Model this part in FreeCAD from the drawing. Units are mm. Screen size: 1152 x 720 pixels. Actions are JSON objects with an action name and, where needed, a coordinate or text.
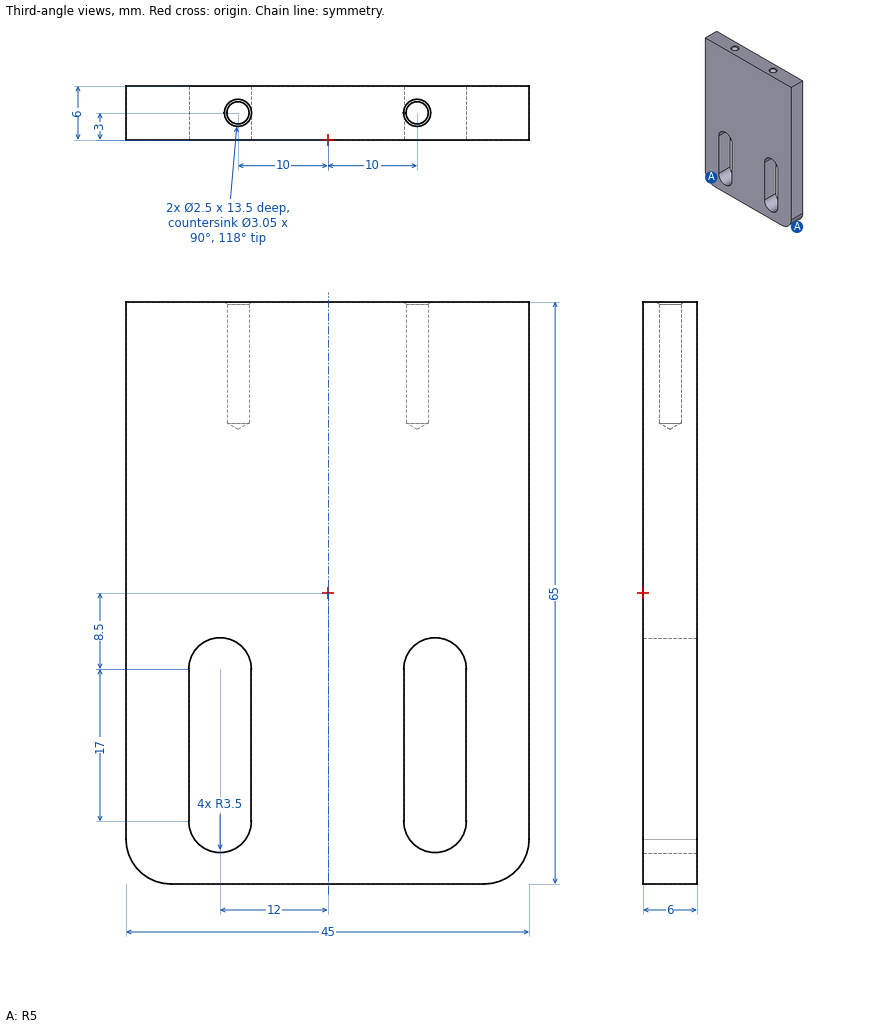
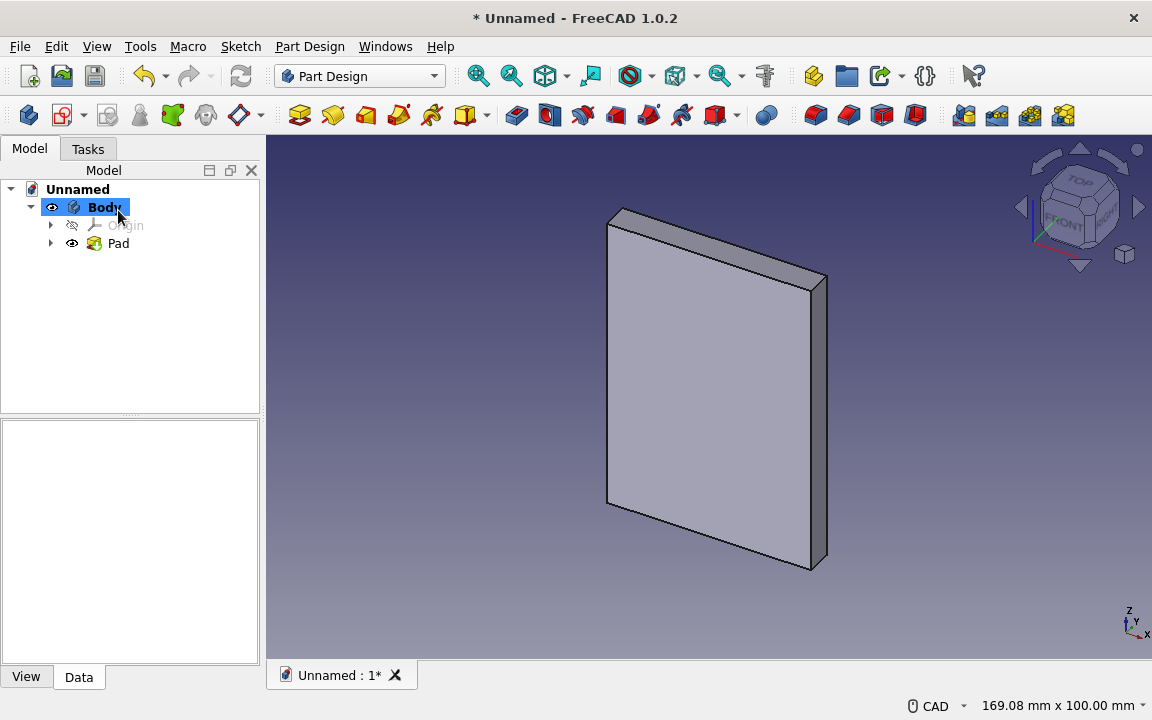
{"action": "key", "text": "4"}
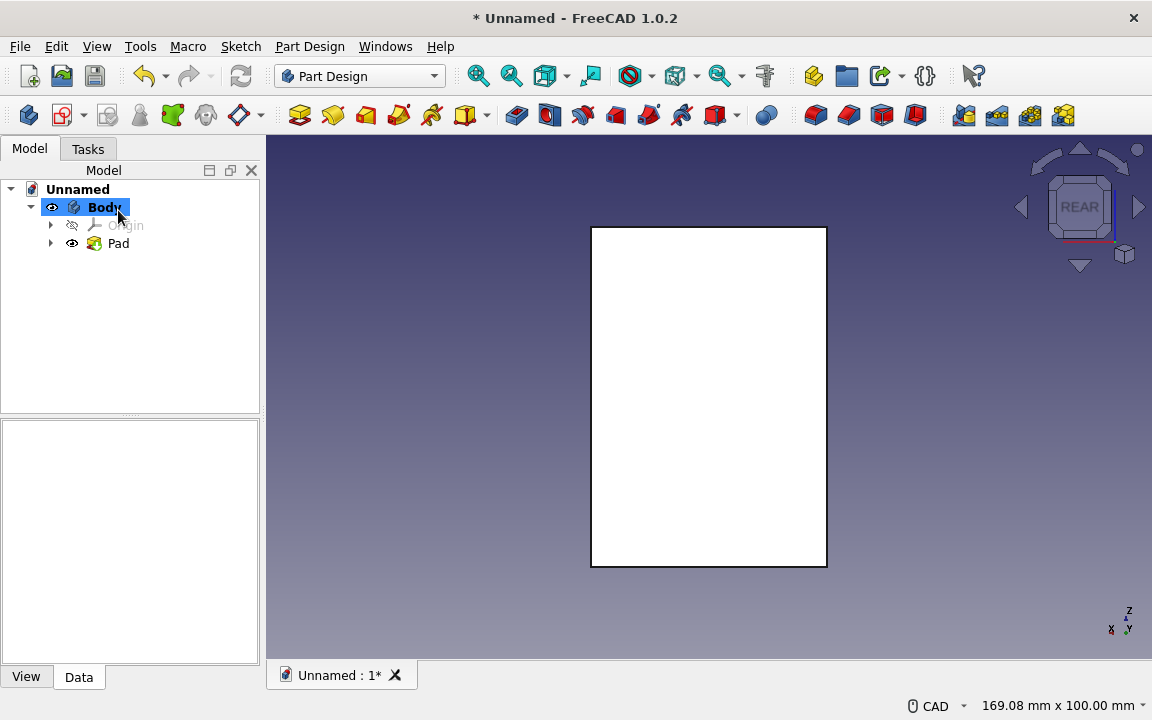
{"action": "left_click", "coordinate": [709, 347]}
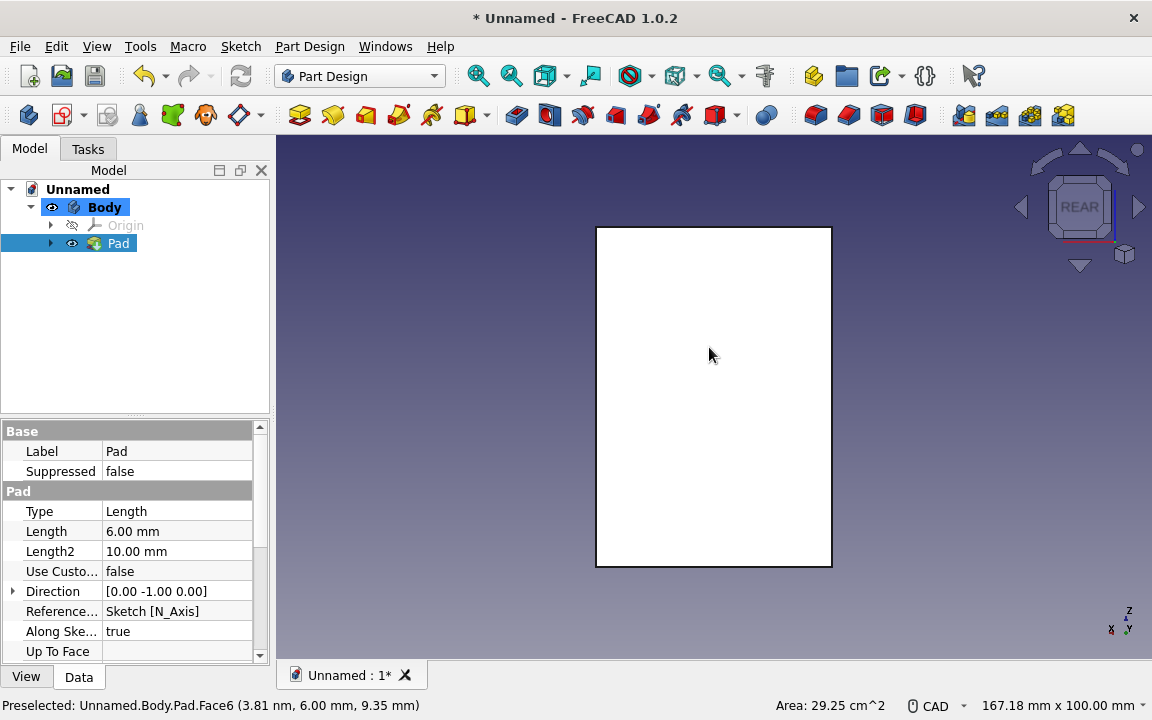
{"action": "left_click", "coordinate": [62, 116]}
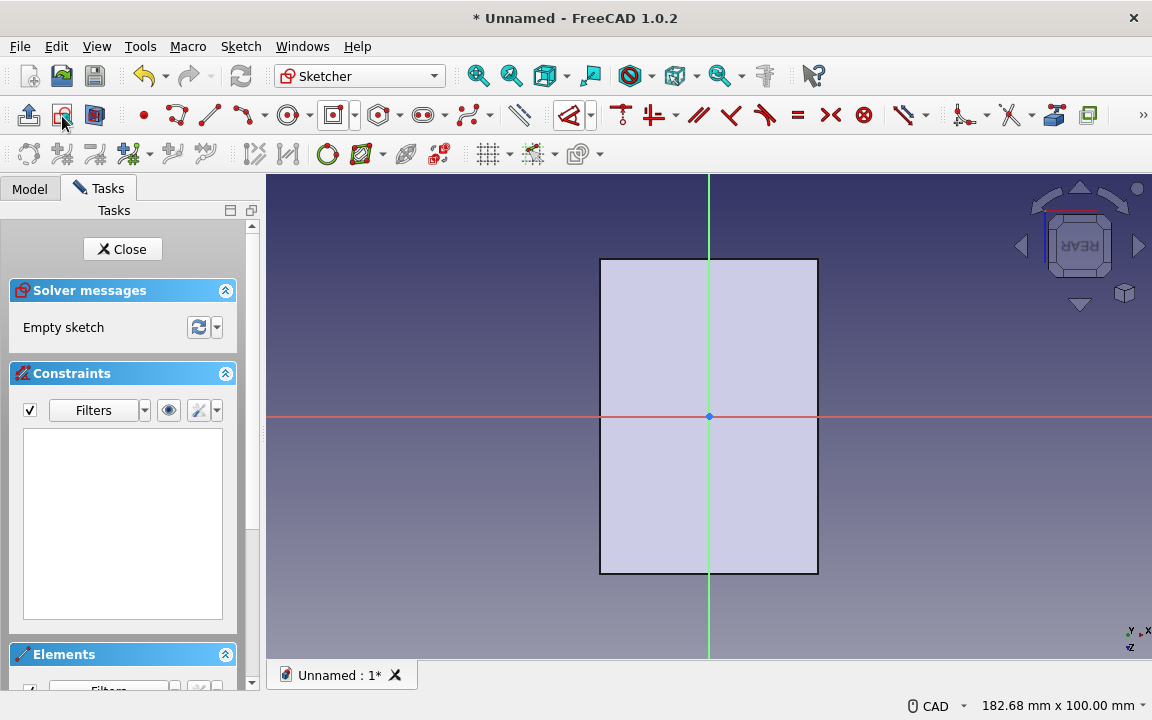
{"action": "scroll", "coordinate": [765, 289], "scroll_direction": "up", "scroll_amount": 4}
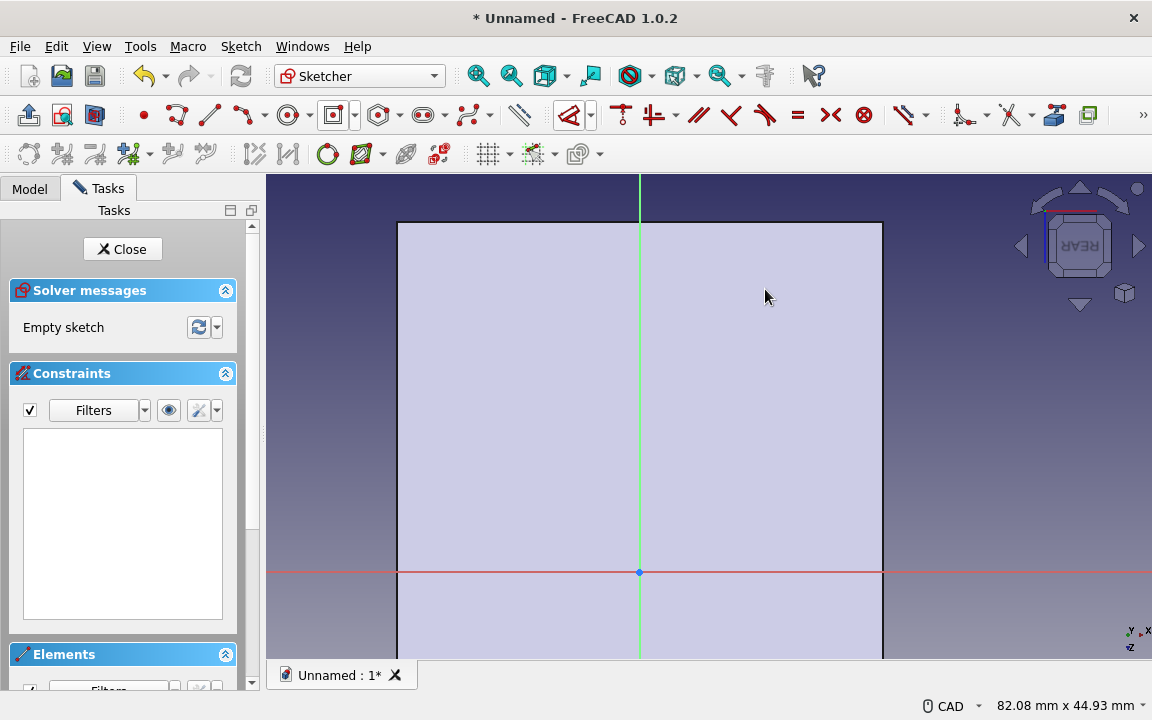
{"action": "key", "text": "g s"}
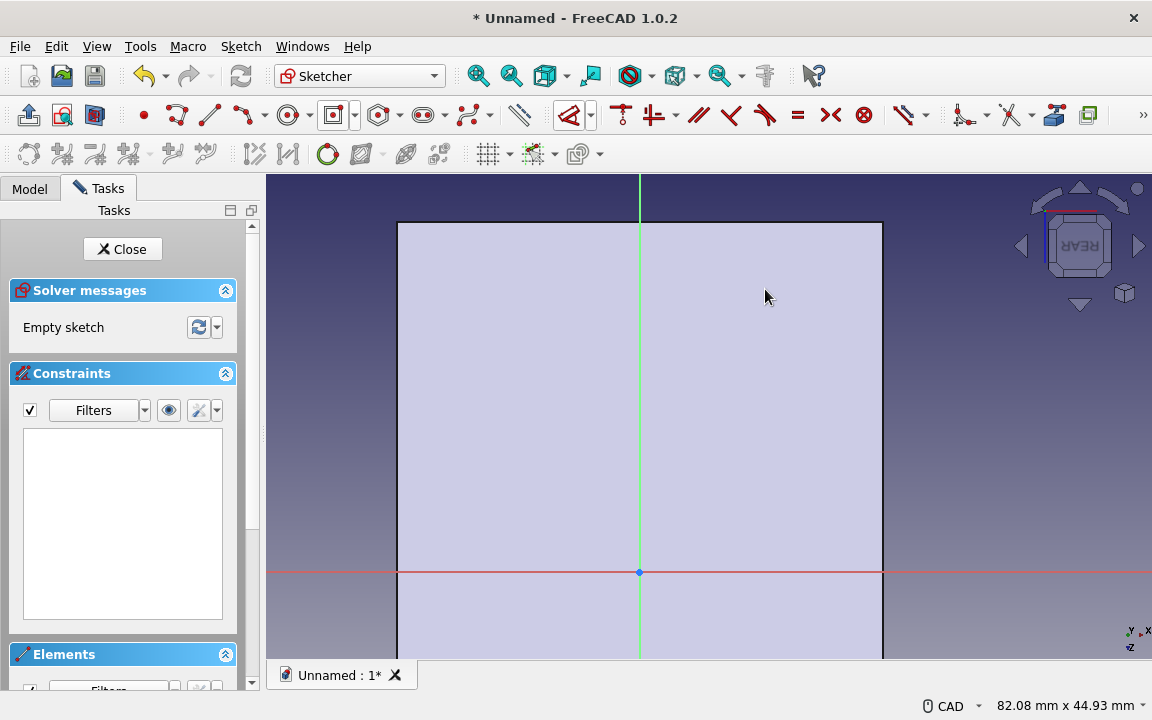
{"action": "left_click", "coordinate": [510, 481]}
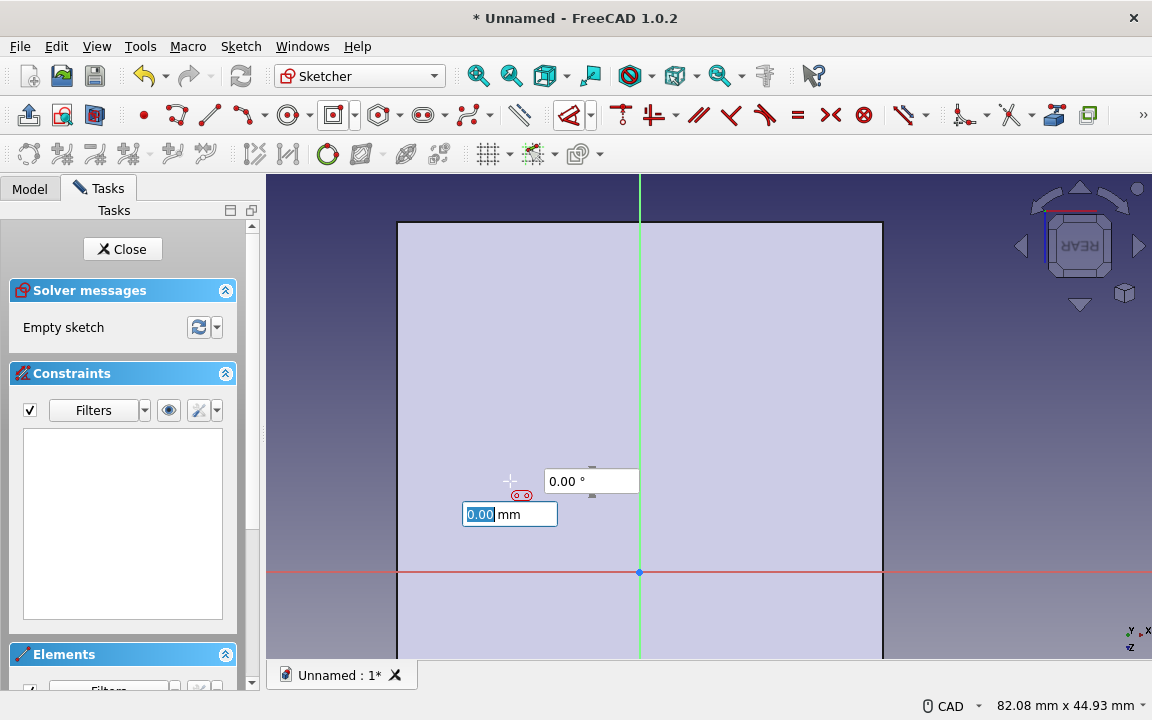
{"action": "left_click", "coordinate": [510, 297]}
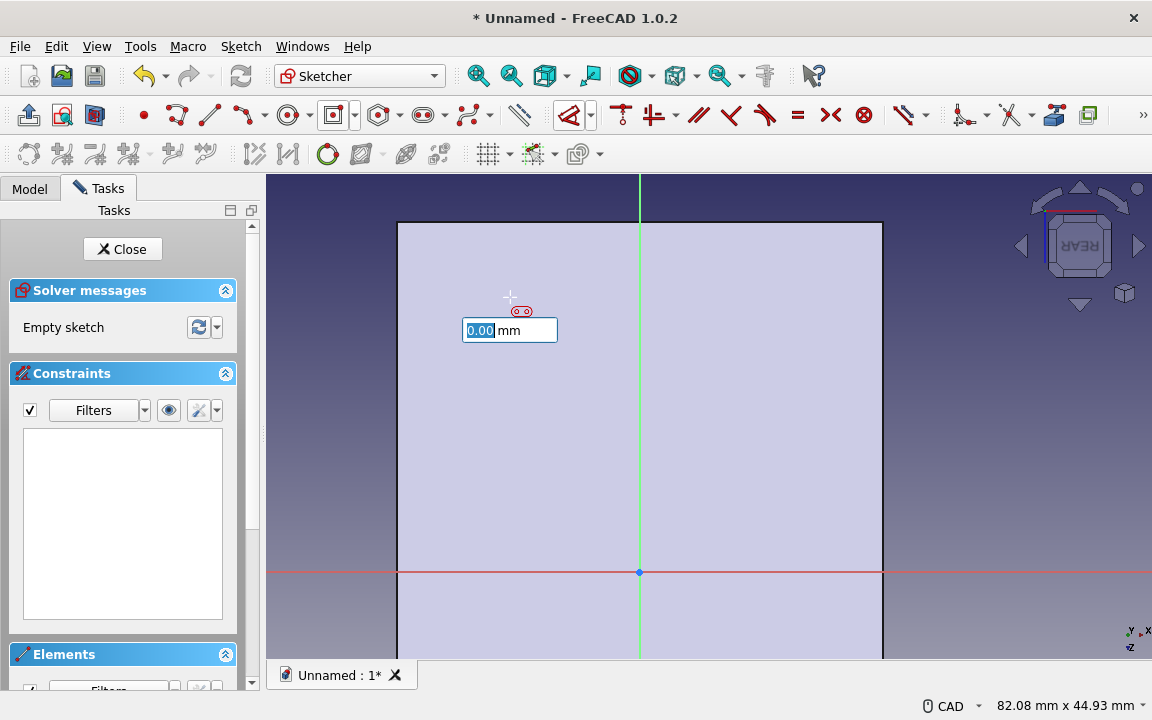
{"action": "left_click", "coordinate": [548, 389]}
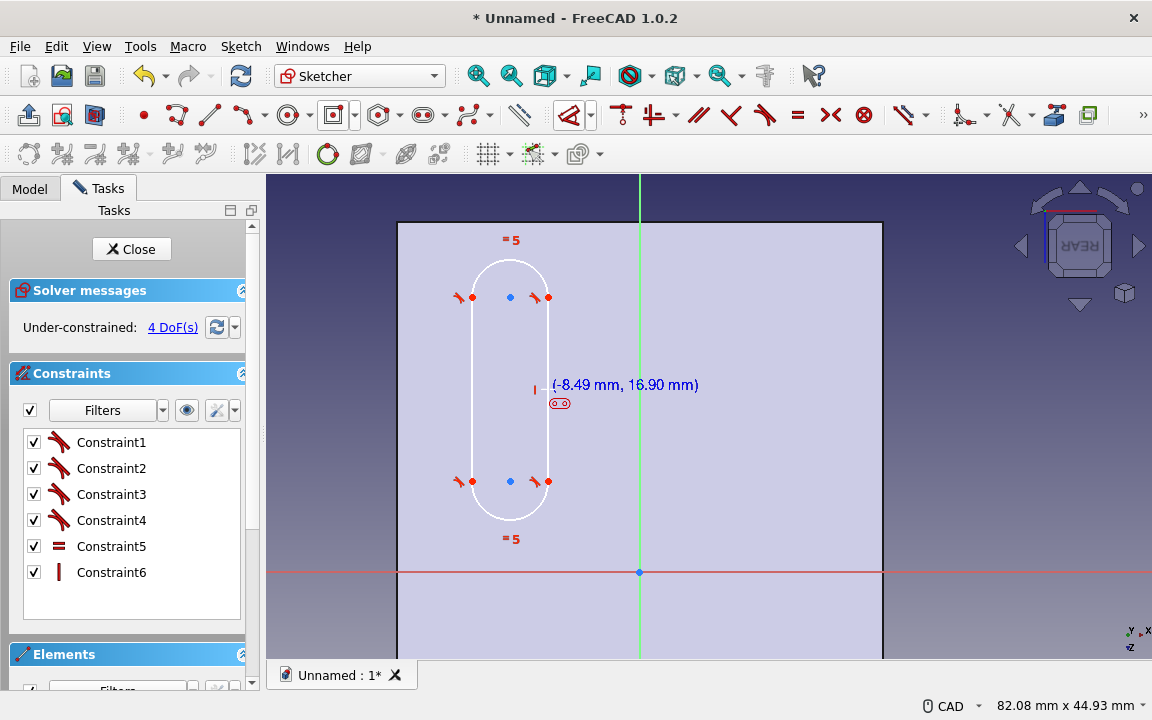
{"action": "left_click", "coordinate": [769, 481]}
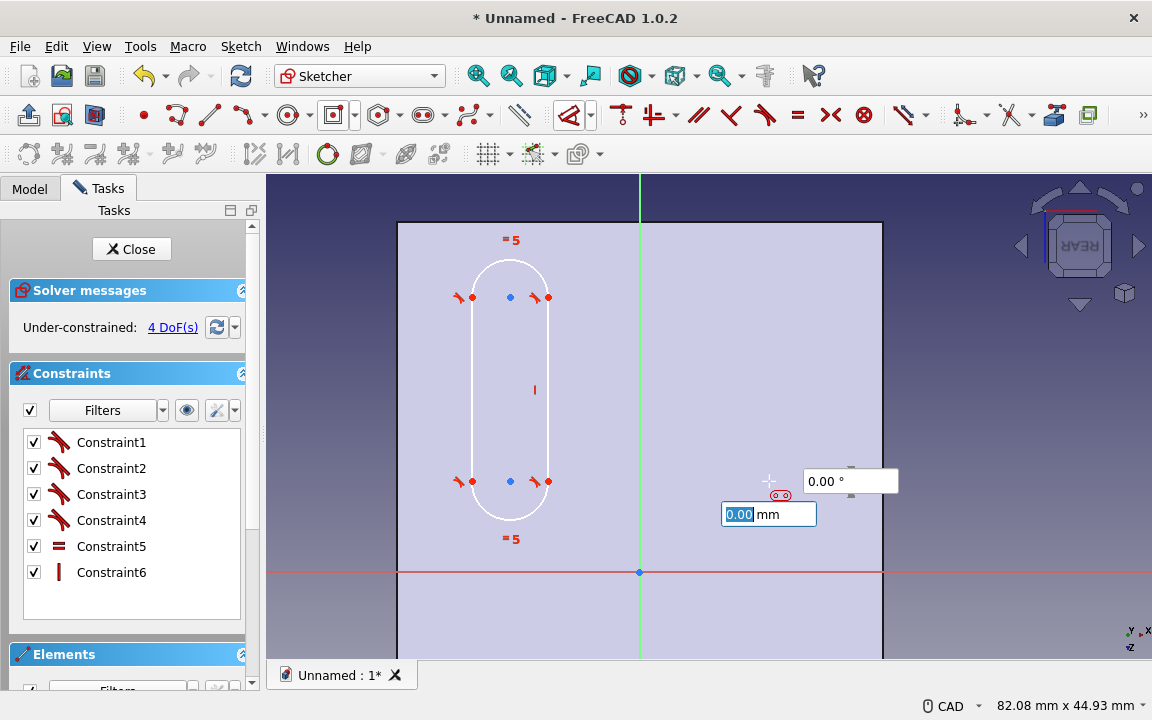
{"action": "left_click", "coordinate": [769, 297]}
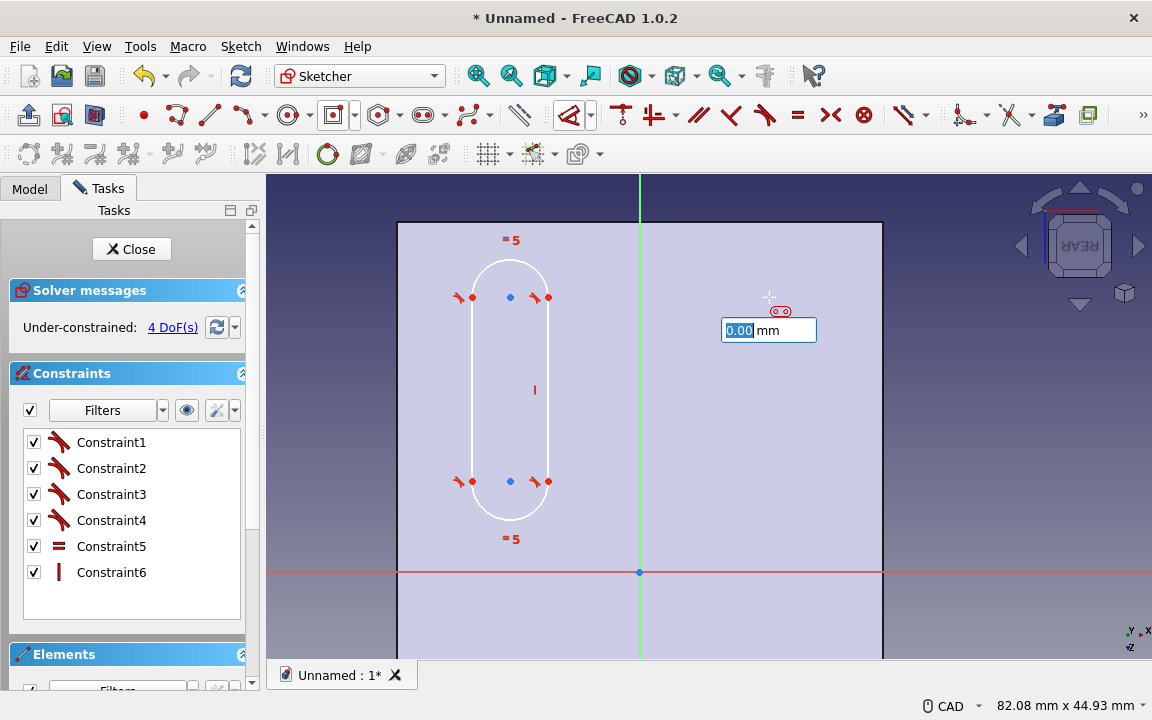
{"action": "left_click", "coordinate": [731, 389]}
{"action": "key", "text": "Escape"}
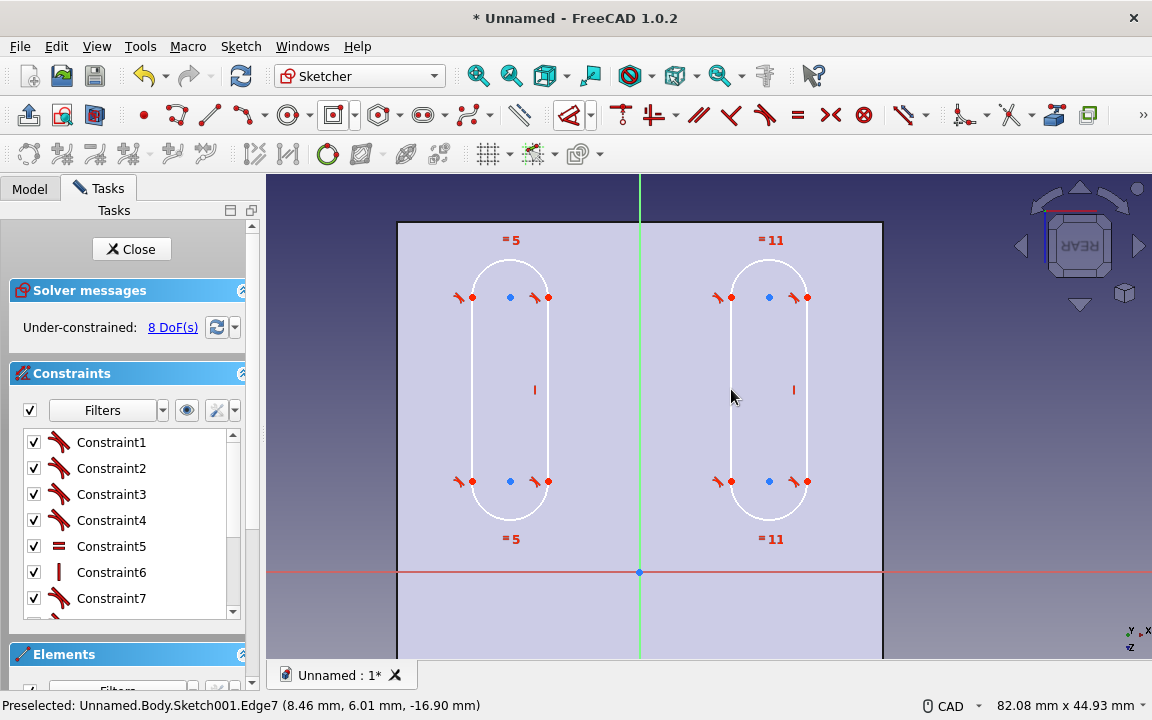
{"action": "left_click", "coordinate": [488, 513]}